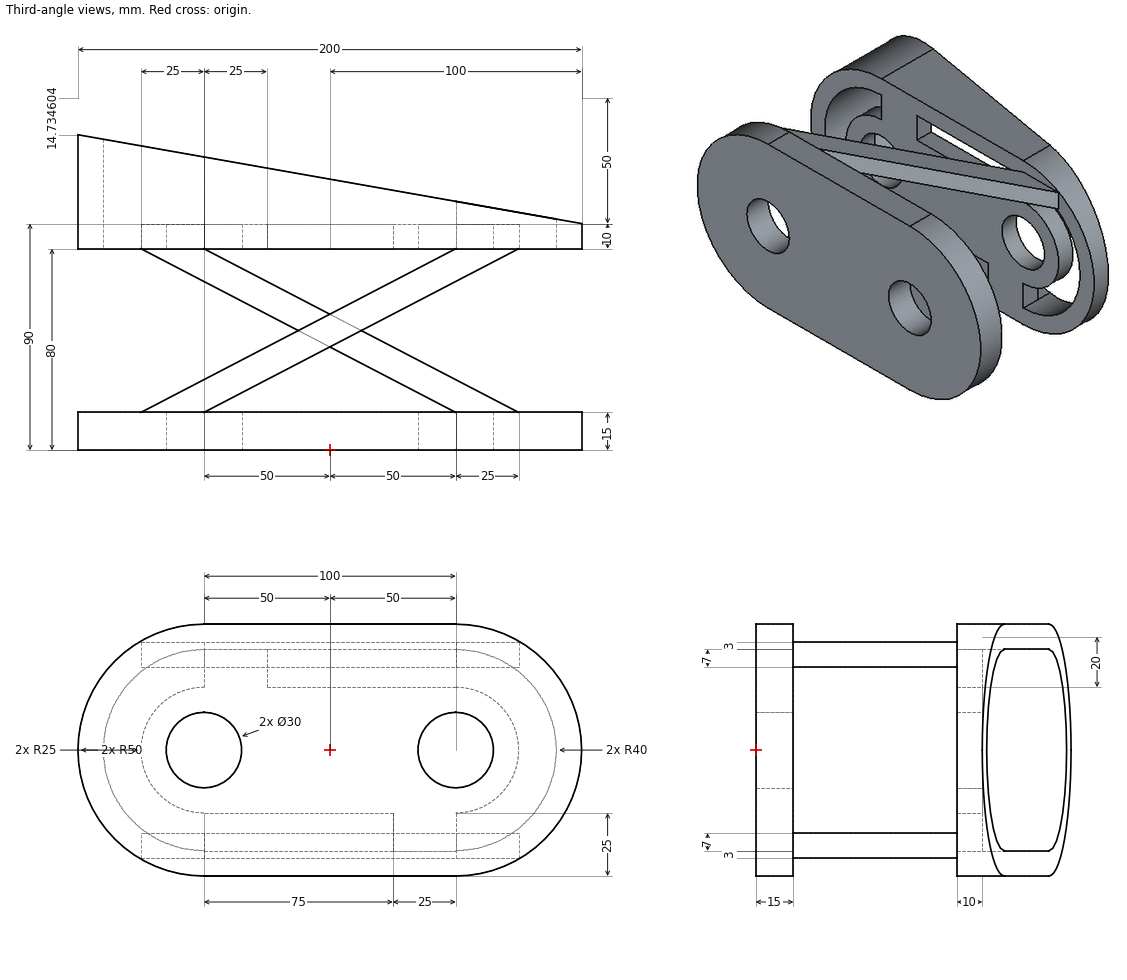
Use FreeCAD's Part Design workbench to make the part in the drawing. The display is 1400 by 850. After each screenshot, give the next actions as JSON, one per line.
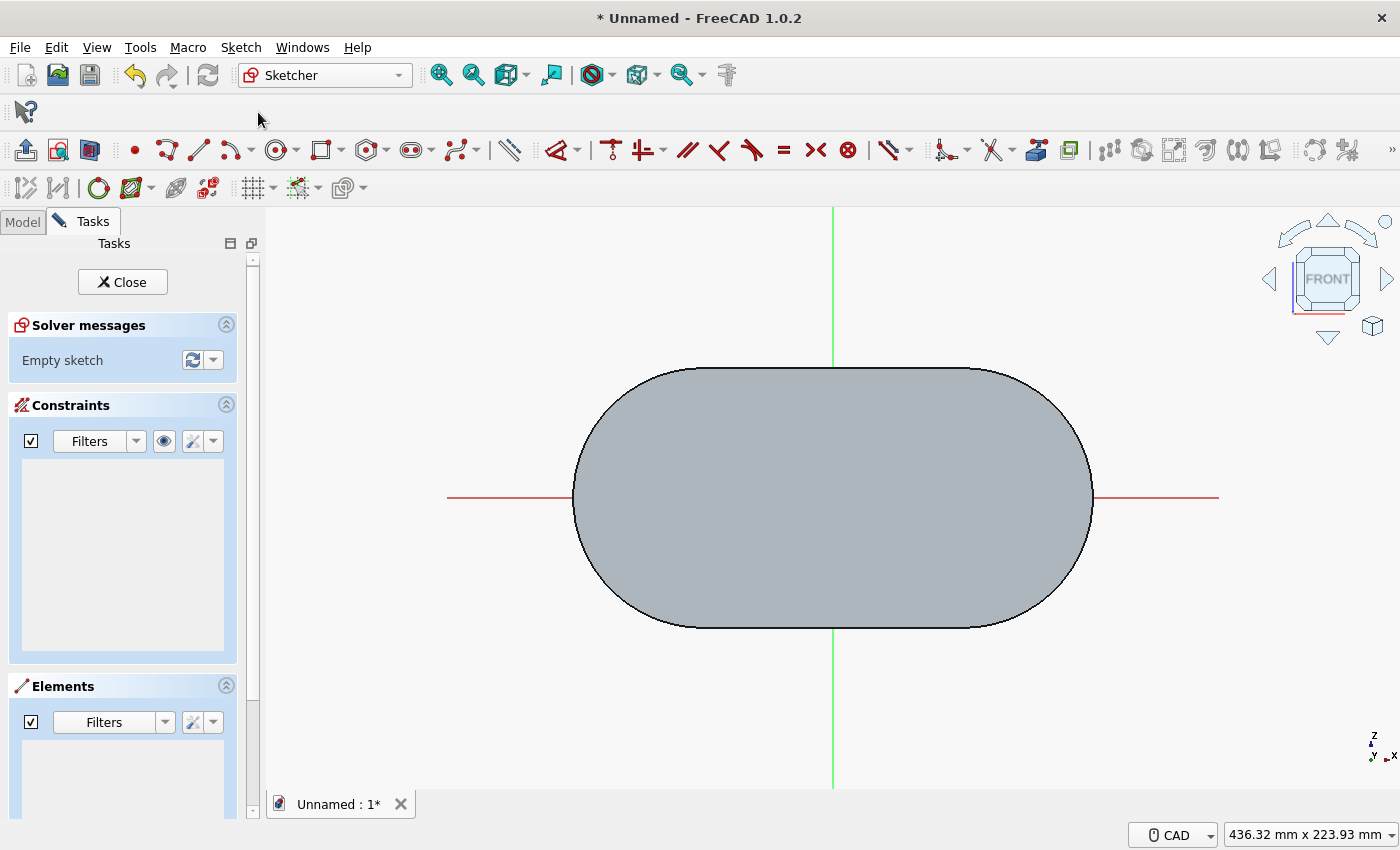
{"action": "scroll", "coordinate": [916, 570], "scroll_direction": "up", "scroll_amount": 3}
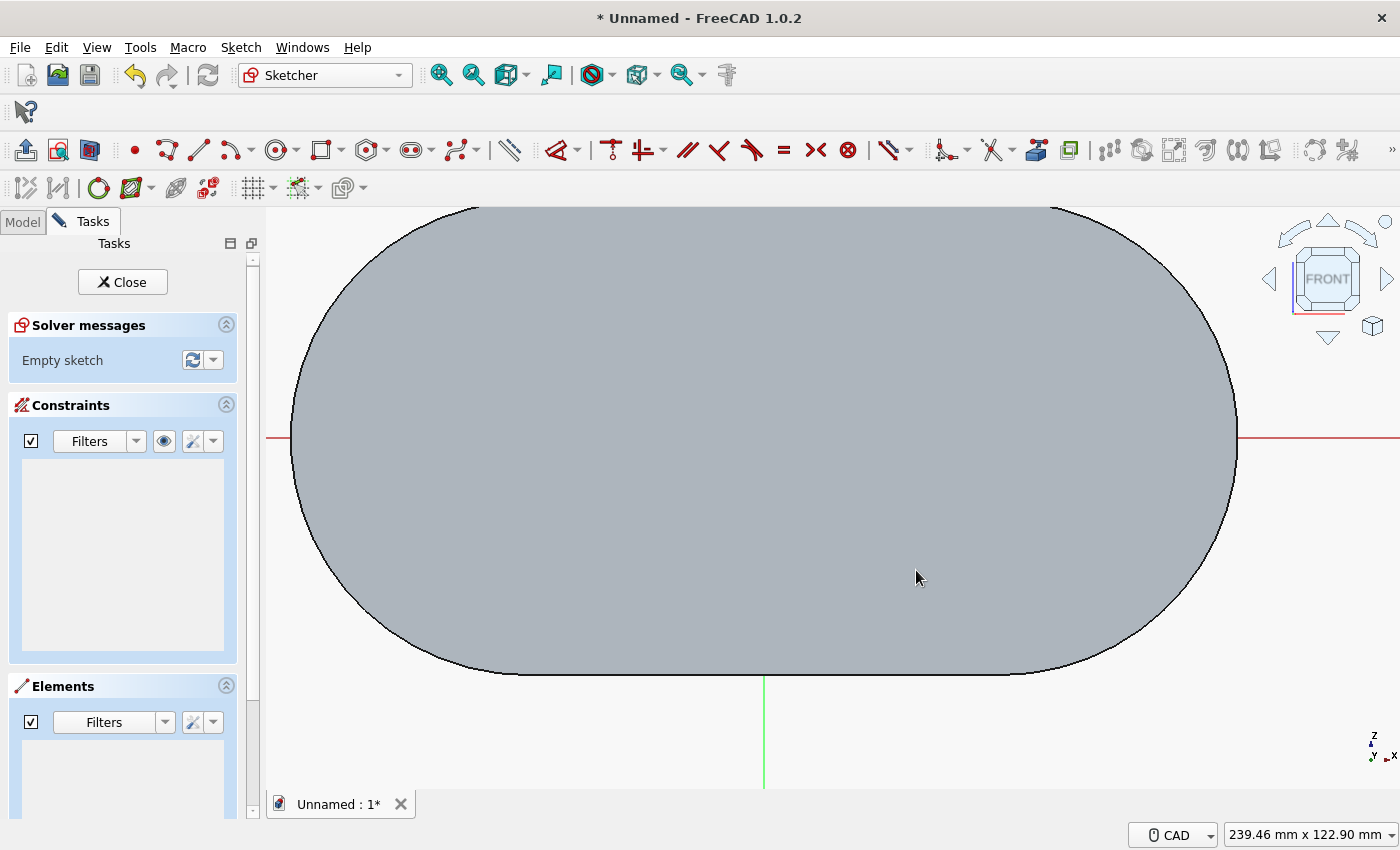
{"action": "left_click", "coordinate": [200, 150]}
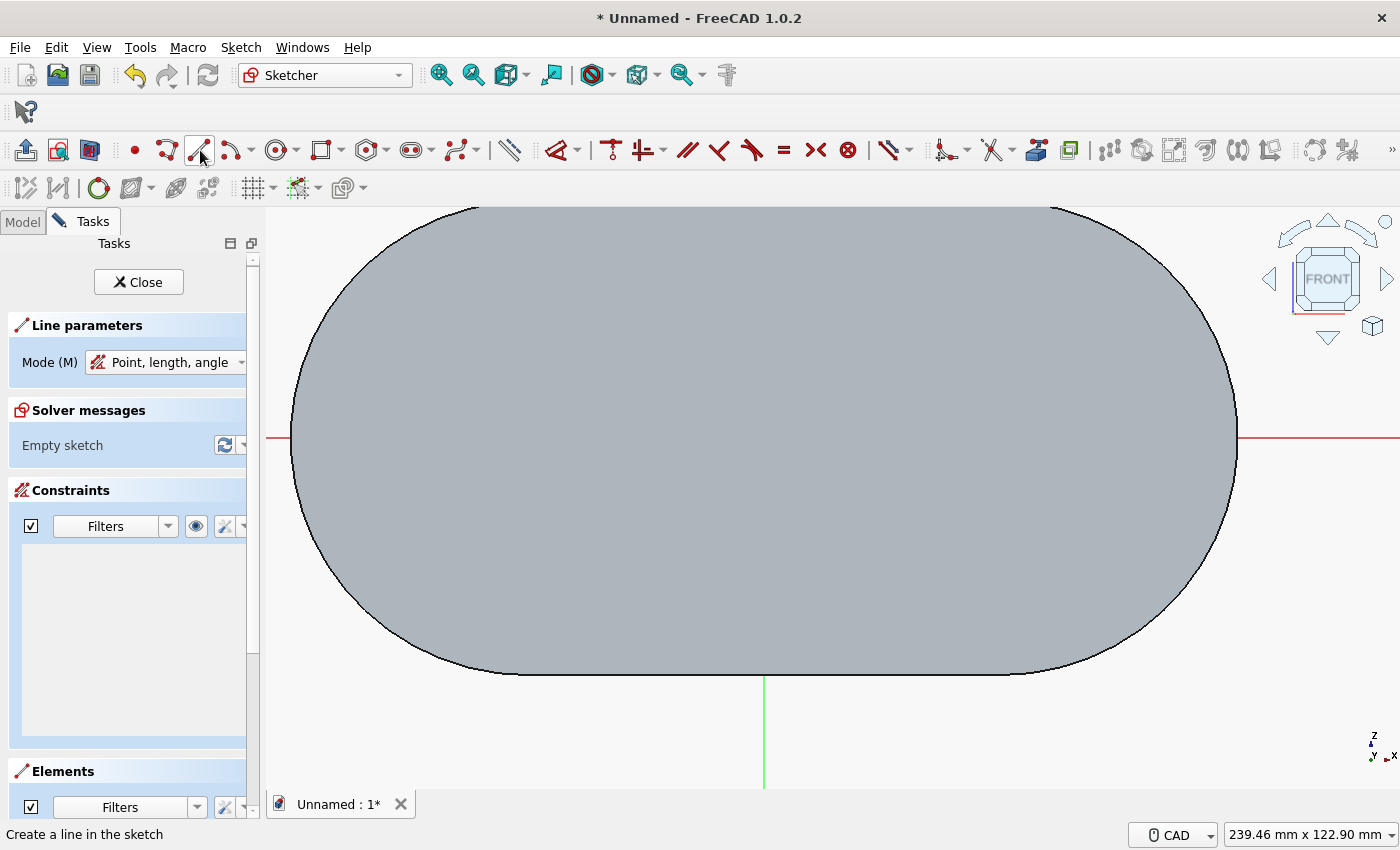
{"action": "left_click", "coordinate": [528, 320]}
{"action": "left_click", "coordinate": [1001, 320]}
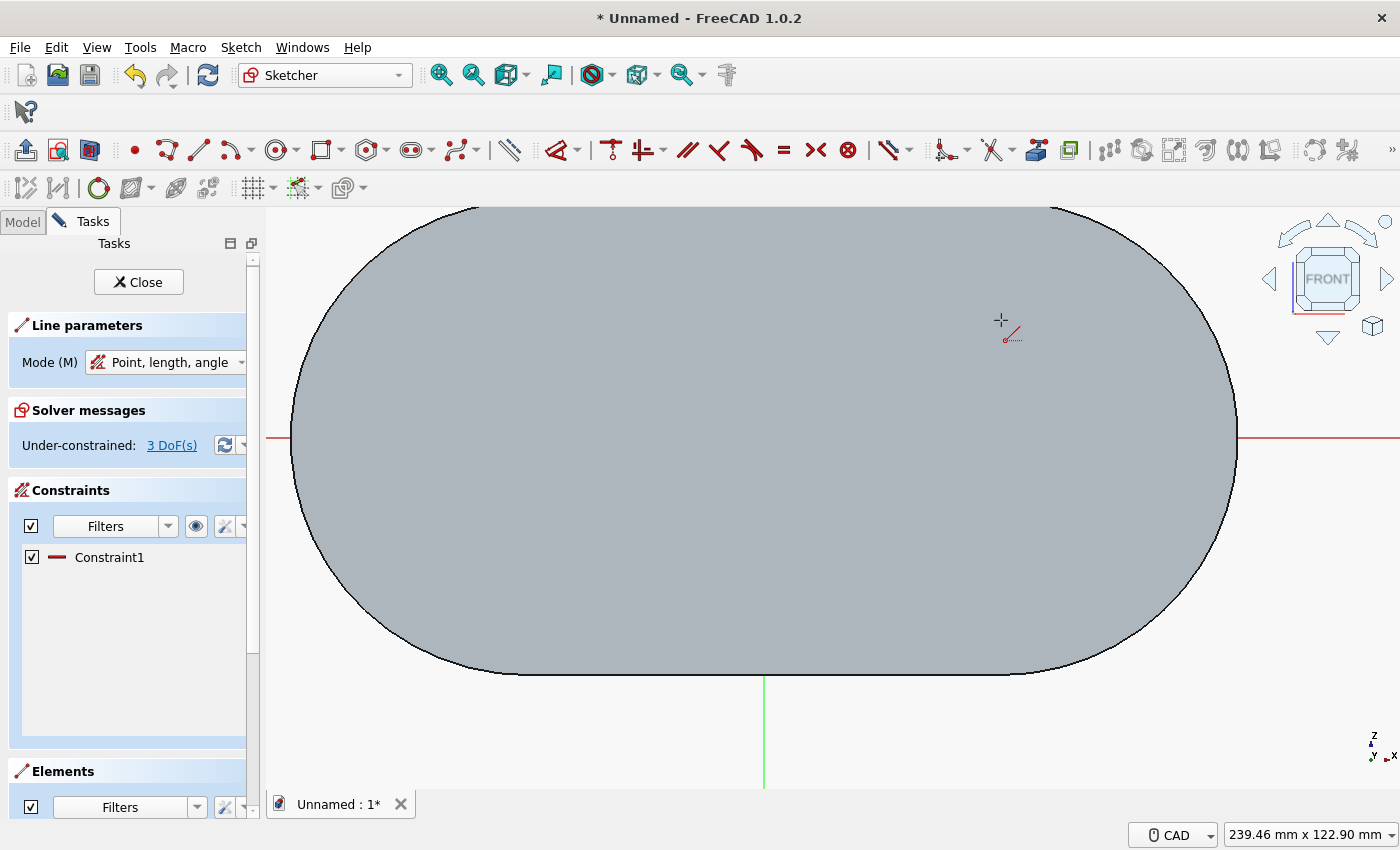
{"action": "left_click", "coordinate": [168, 150]}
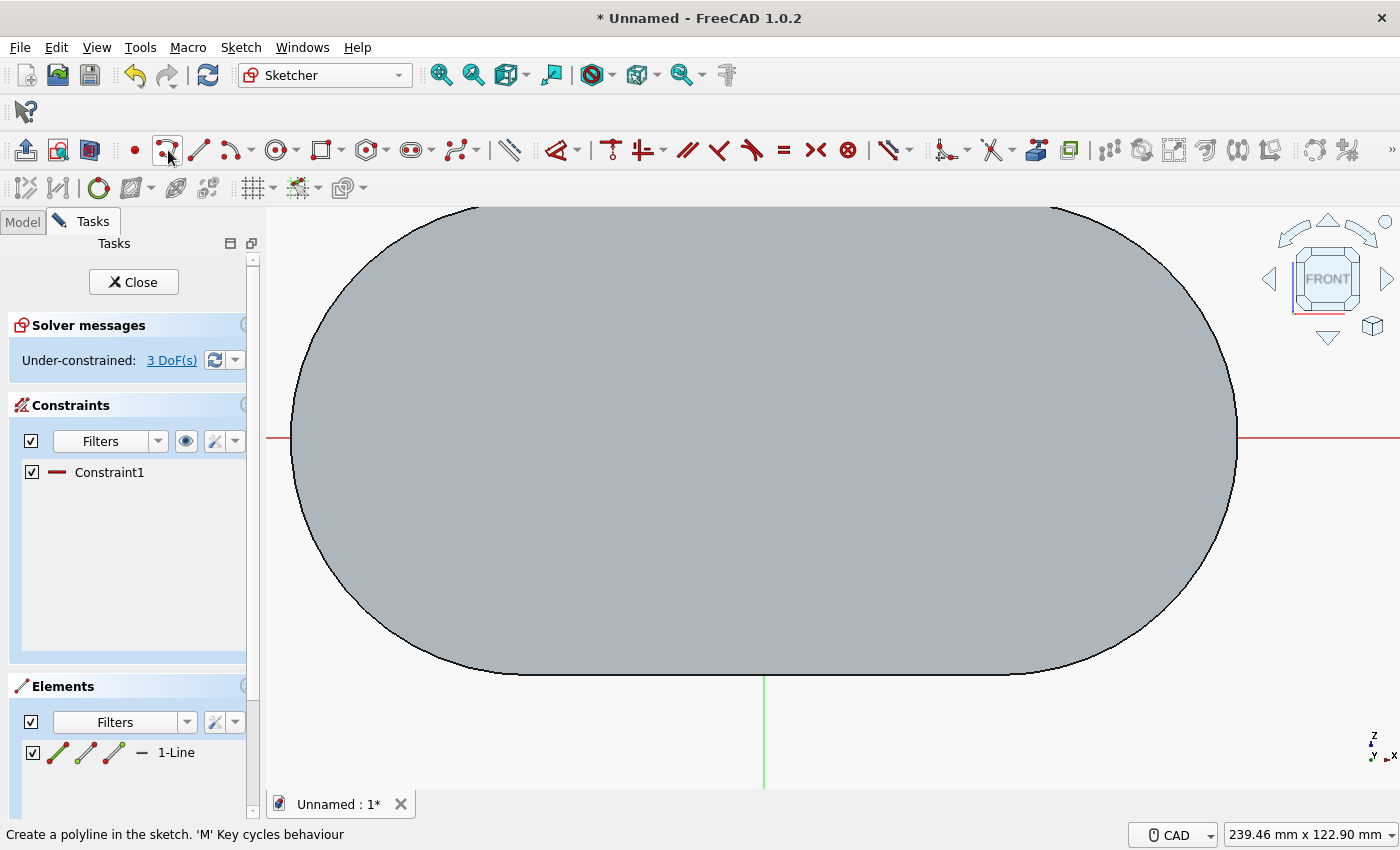
{"action": "left_click", "coordinate": [1001, 557]}
{"action": "left_click", "coordinate": [1001, 675]}
{"action": "left_click", "coordinate": [883, 675]}
{"action": "left_click", "coordinate": [883, 557]}
{"action": "left_click", "coordinate": [528, 557]}
{"action": "right_click", "coordinate": [528, 557]}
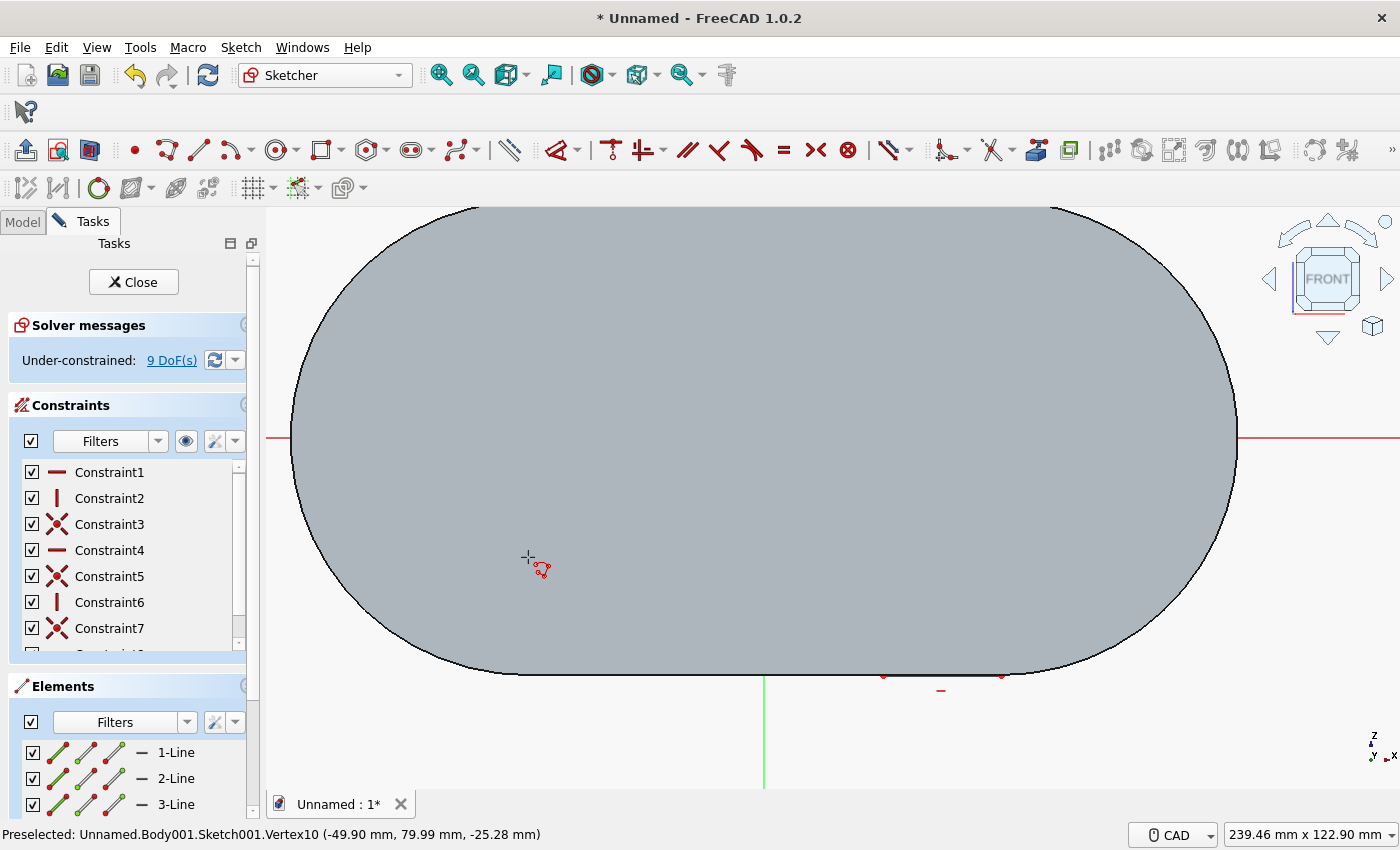
{"action": "key", "text": "g 3 a"}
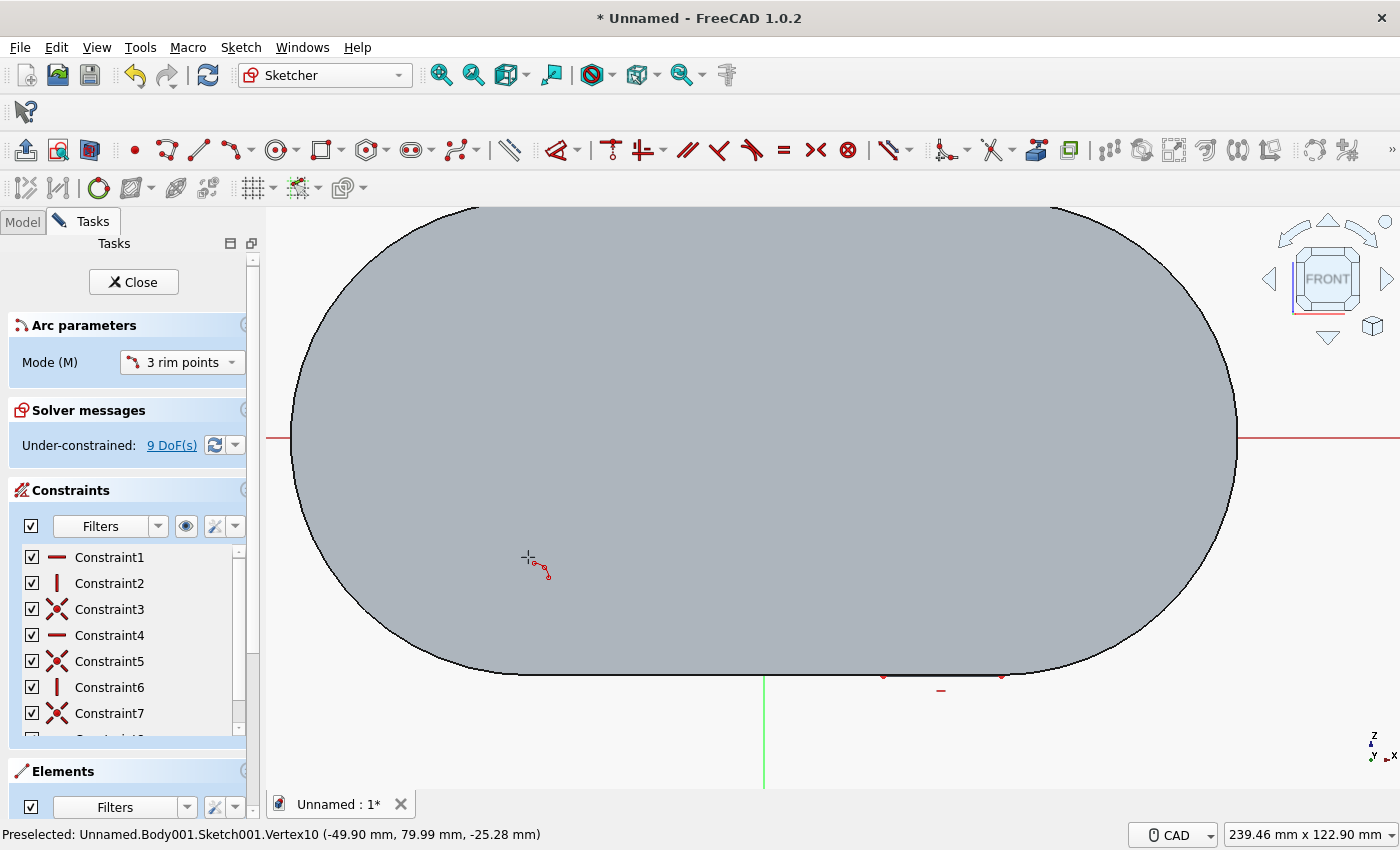
{"action": "left_click", "coordinate": [1001, 321]}
{"action": "left_click", "coordinate": [1001, 558]}
{"action": "left_click", "coordinate": [1114, 475]}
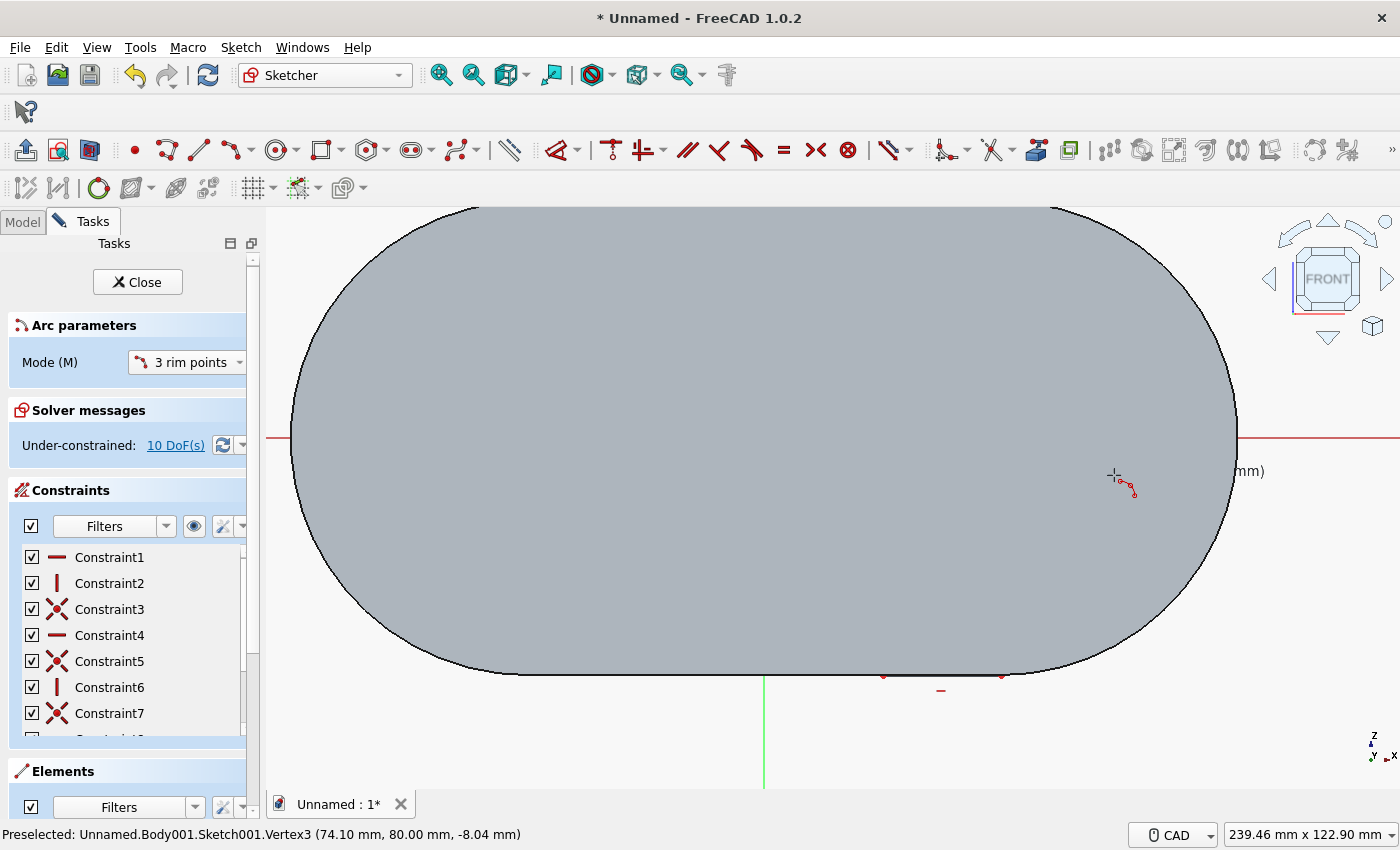
{"action": "left_click", "coordinate": [528, 558]}
{"action": "left_click", "coordinate": [528, 321]}
{"action": "left_click", "coordinate": [415, 402]}
{"action": "key", "text": "Escape"}